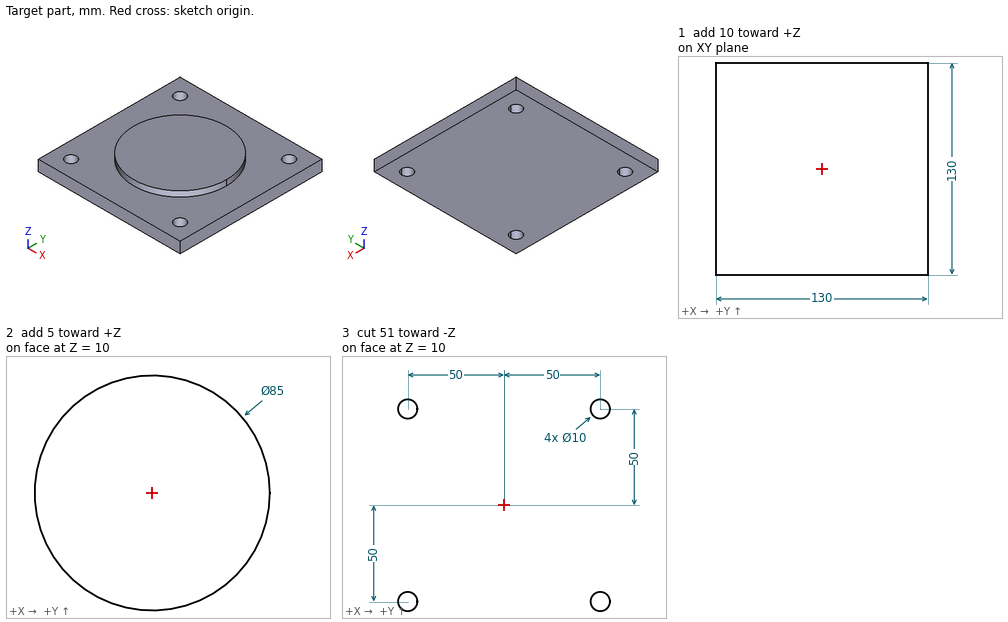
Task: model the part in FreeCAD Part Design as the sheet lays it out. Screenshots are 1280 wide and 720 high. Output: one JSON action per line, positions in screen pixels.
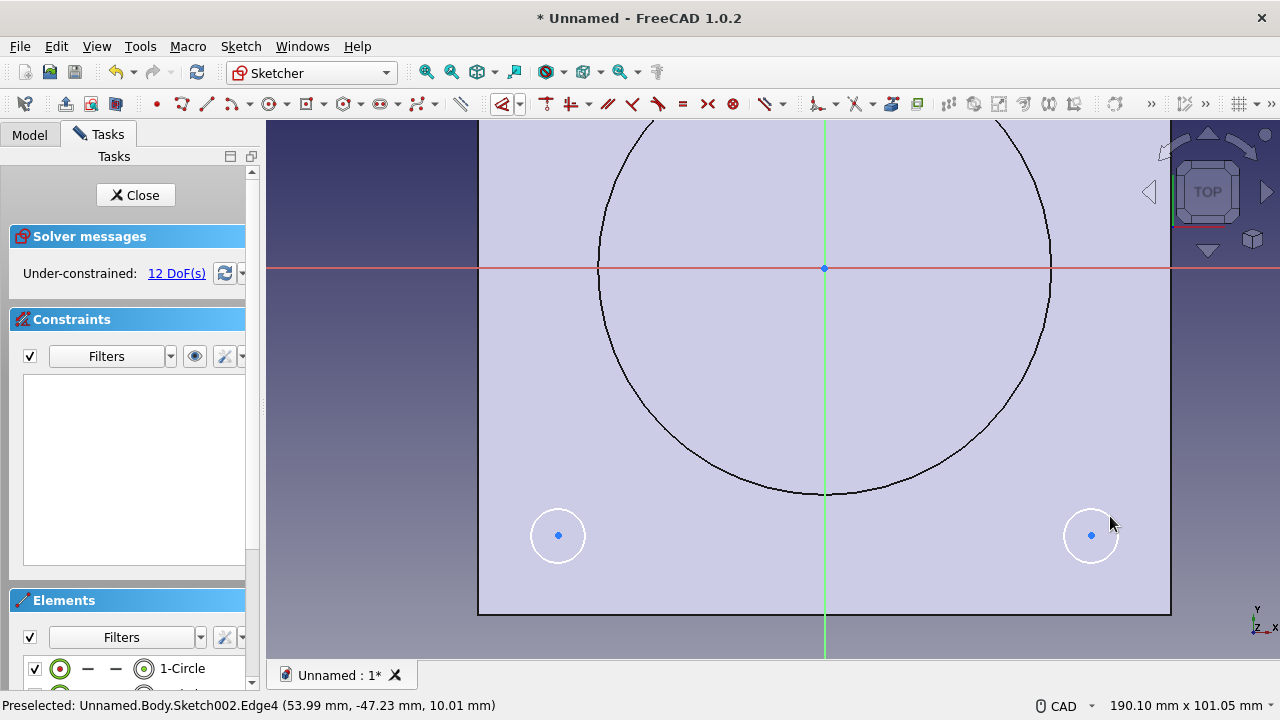
{"action": "scroll", "coordinate": [558, 537], "scroll_direction": "down", "scroll_amount": 3}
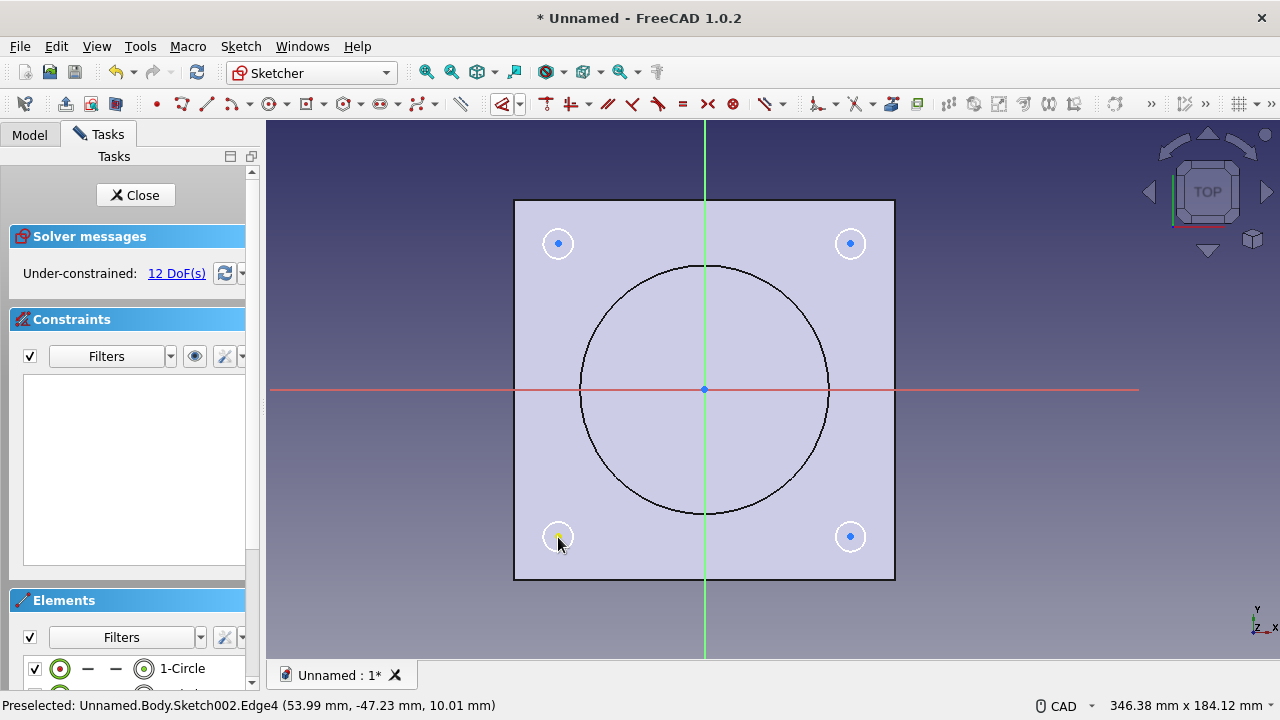
{"action": "left_click", "coordinate": [861, 234]}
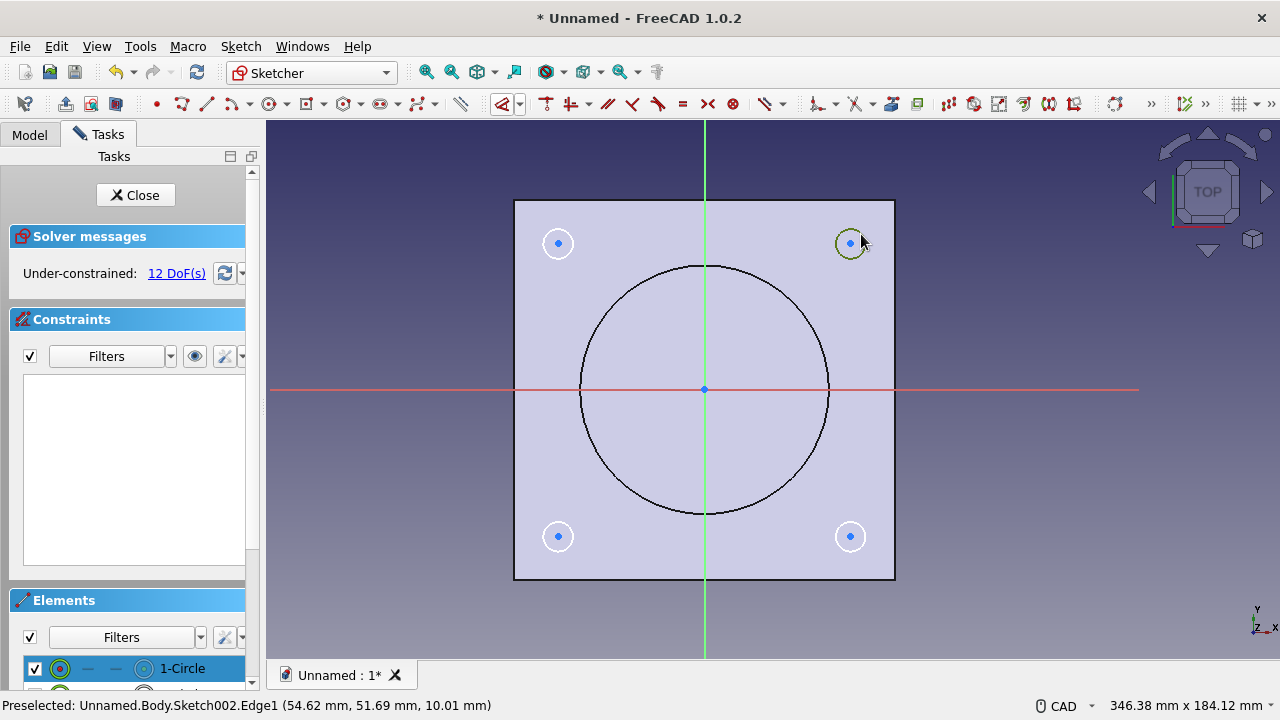
{"action": "left_click", "coordinate": [569, 234]}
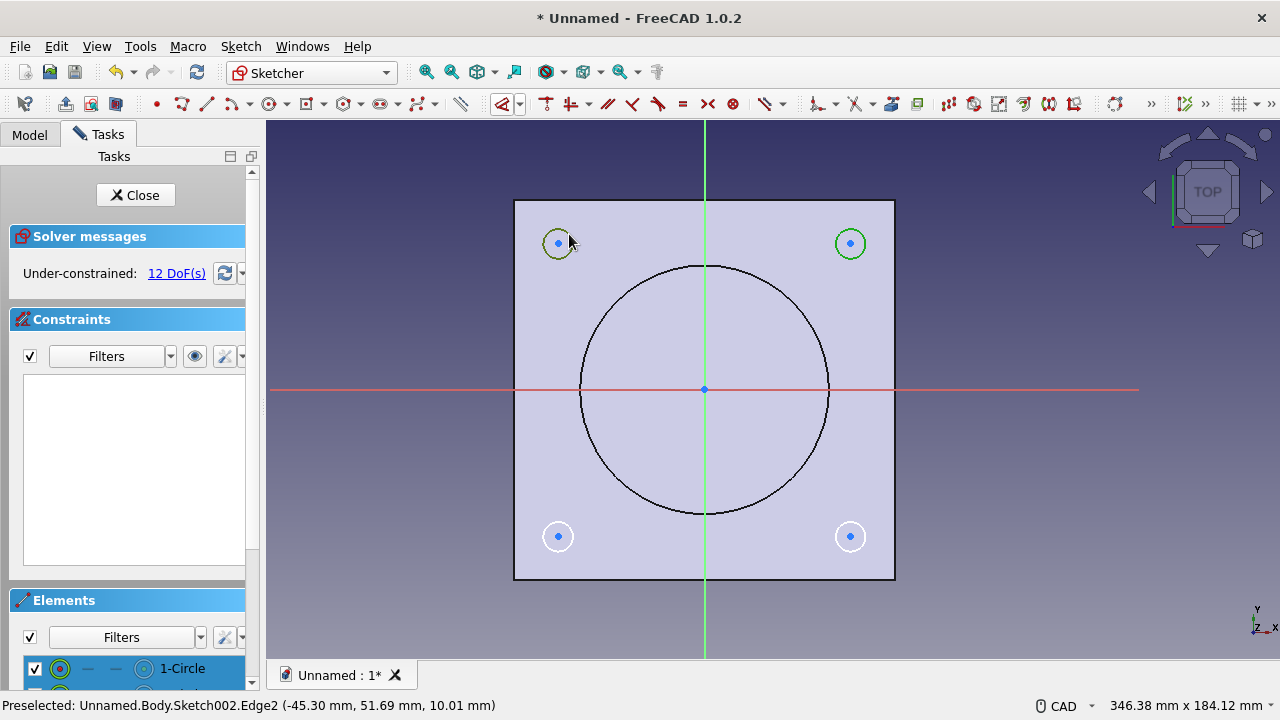
{"action": "left_click", "coordinate": [569, 526]}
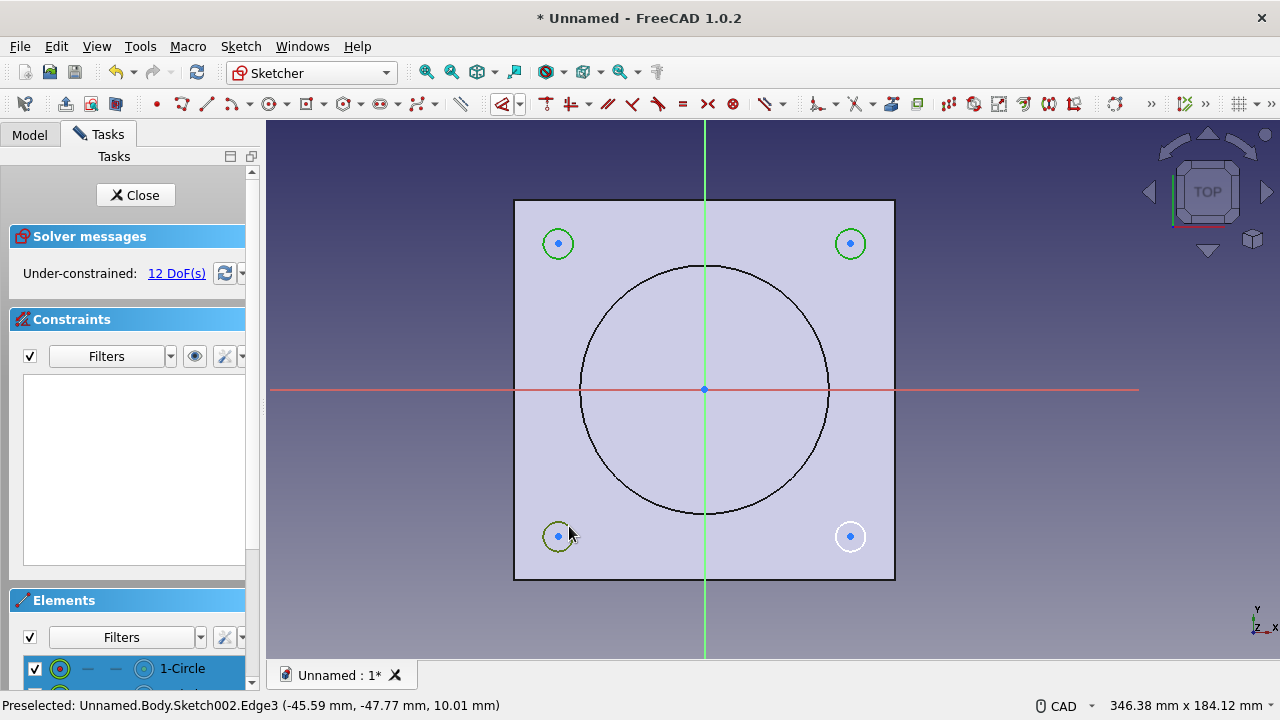
{"action": "left_click", "coordinate": [861, 526]}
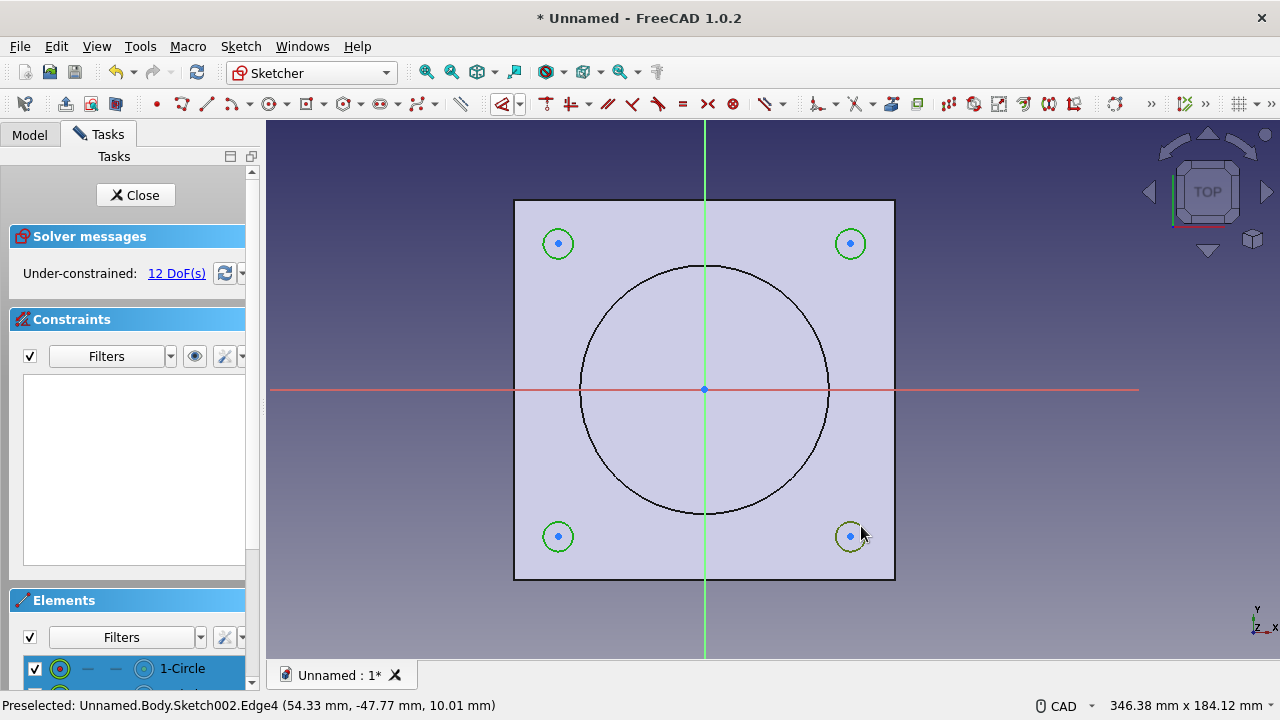
{"action": "left_click", "coordinate": [683, 104]}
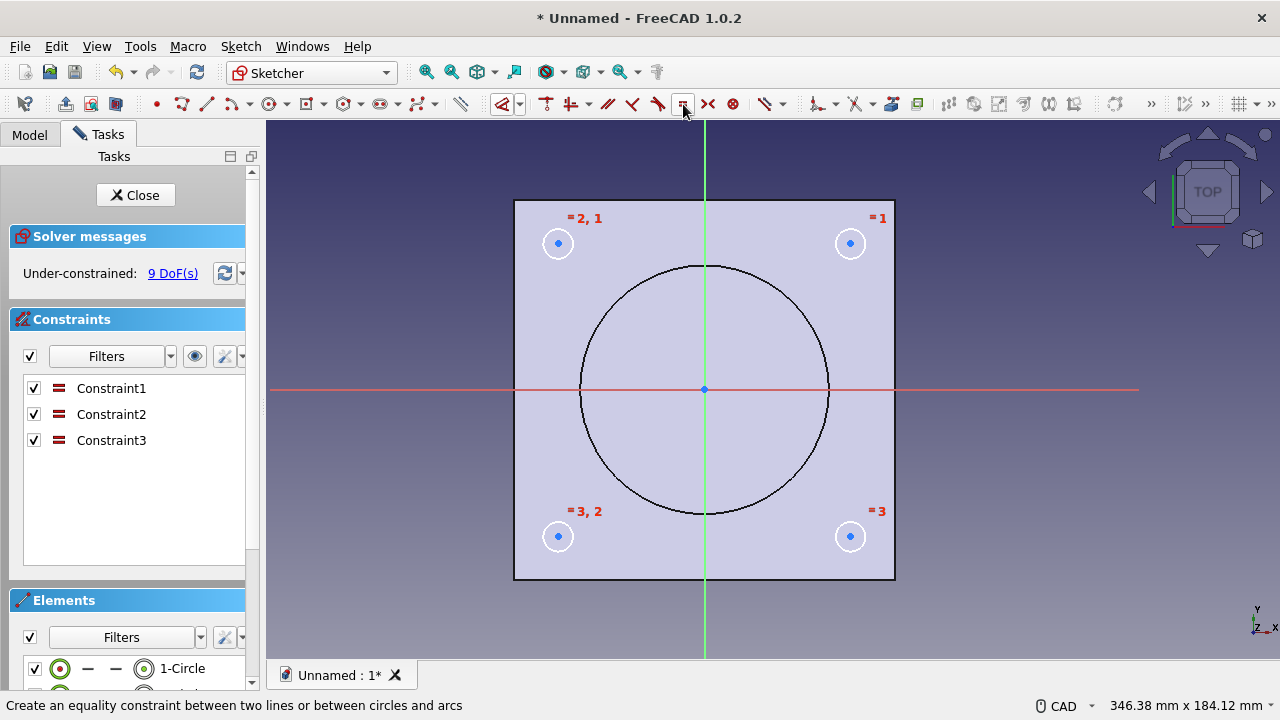
{"action": "left_click", "coordinate": [851, 244]}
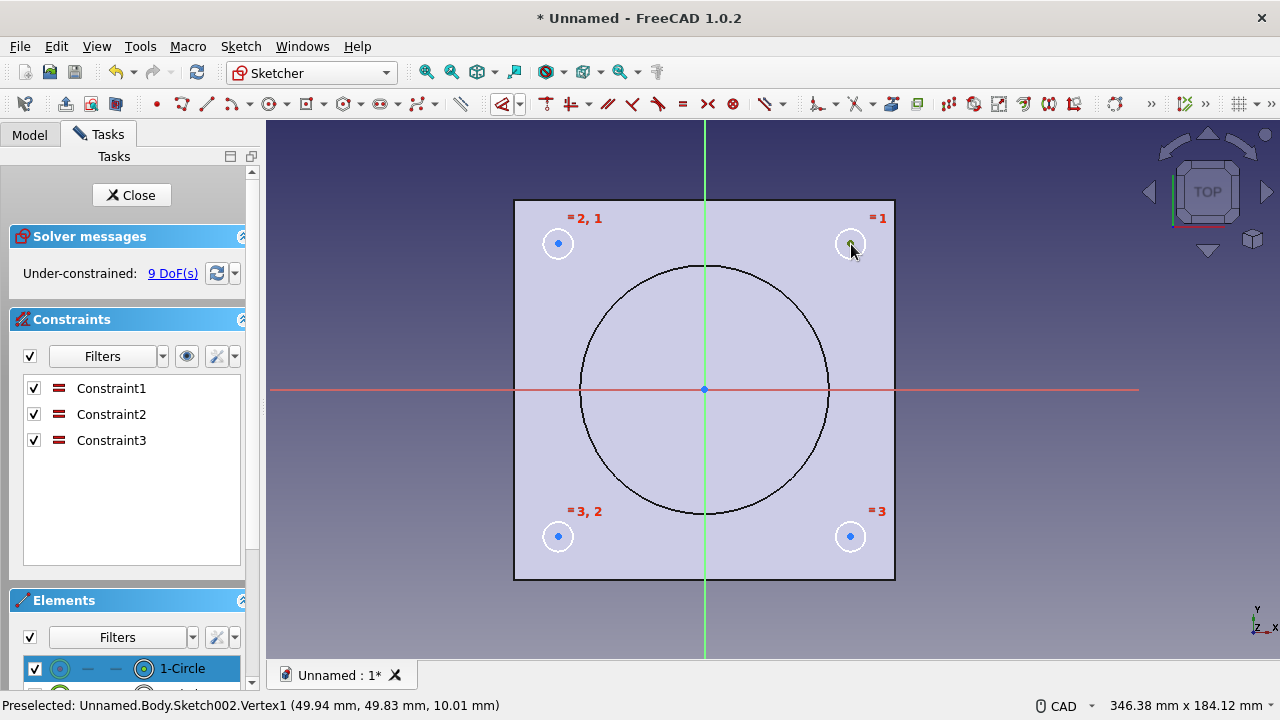
{"action": "left_click", "coordinate": [558, 244]}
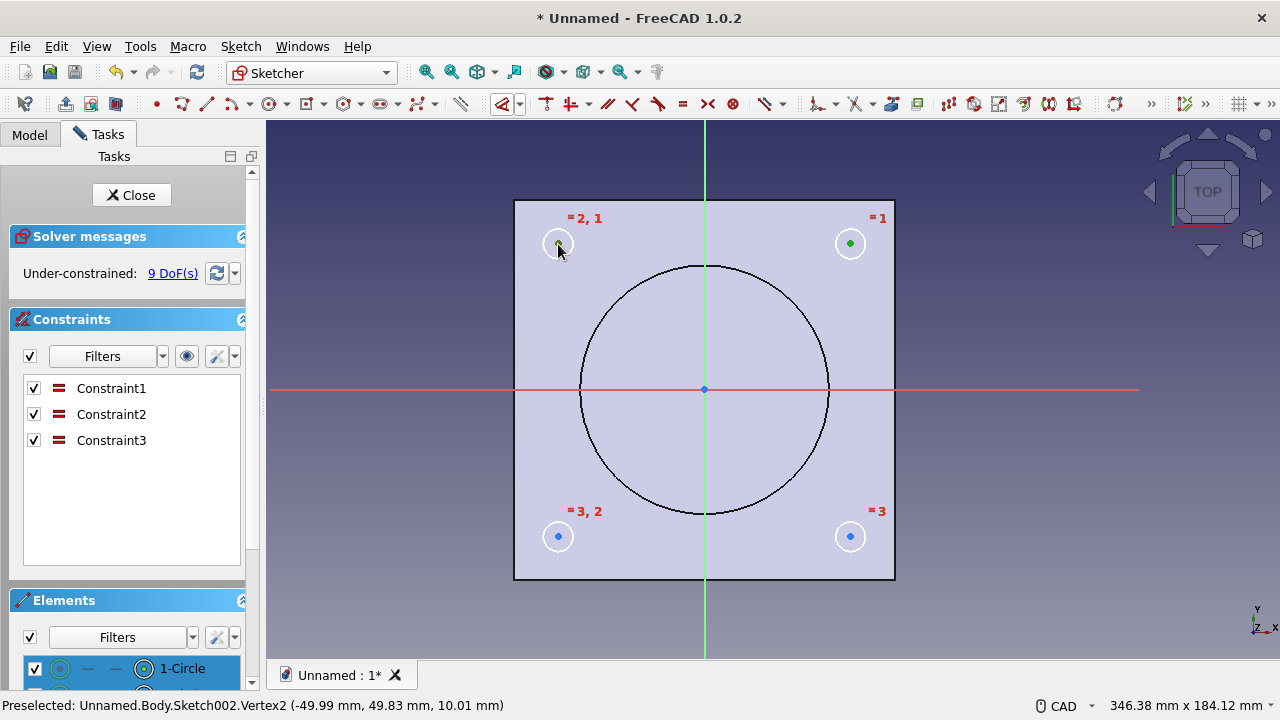
{"action": "key", "text": "h"}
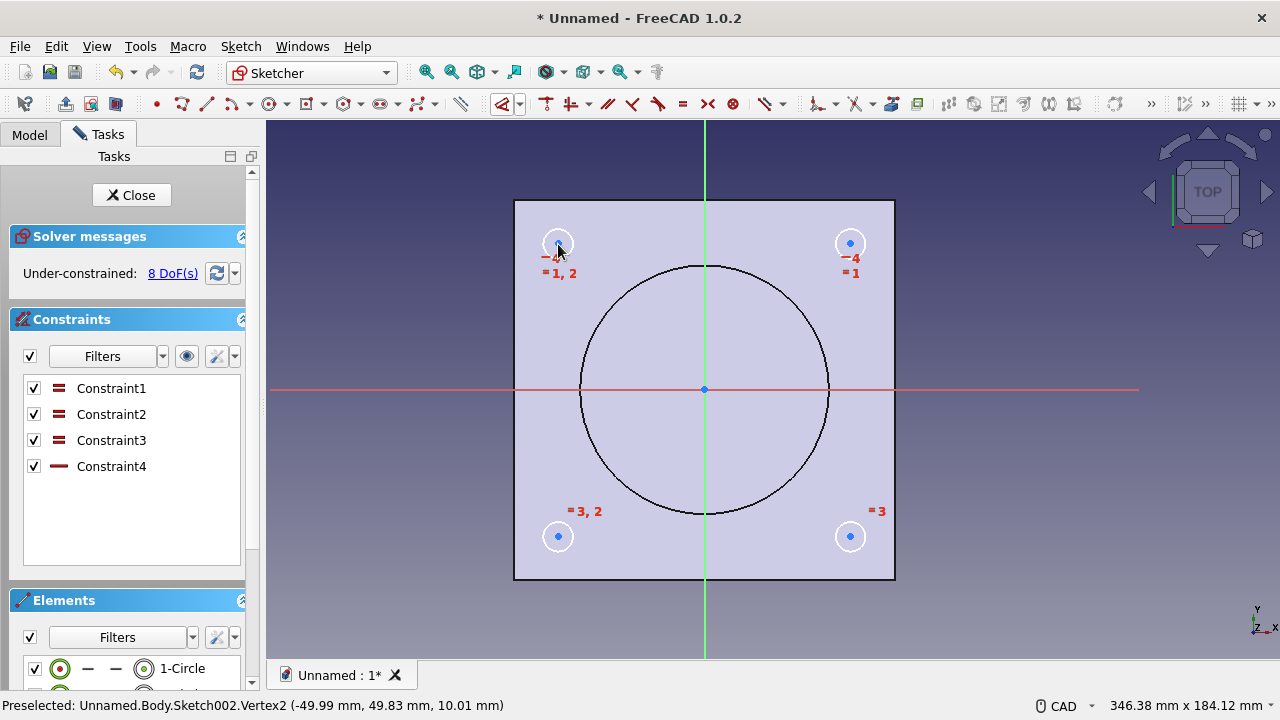
{"action": "left_click", "coordinate": [558, 244]}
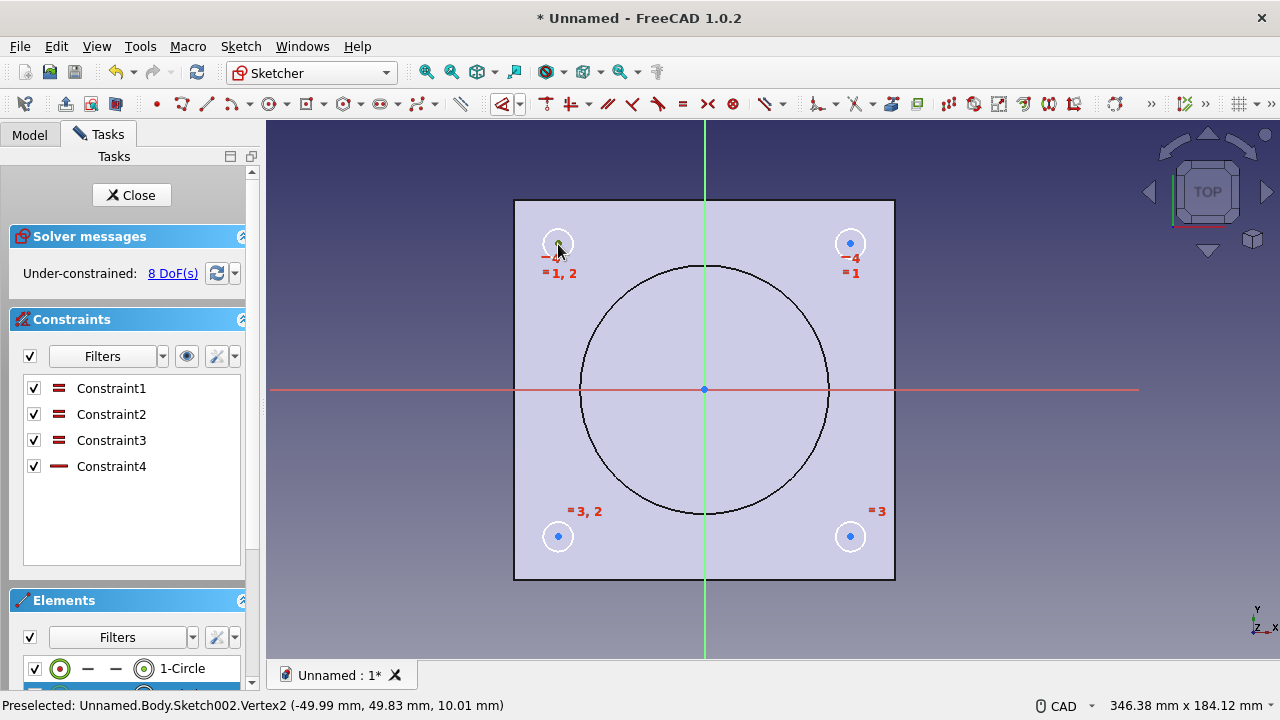
{"action": "left_click", "coordinate": [558, 537]}